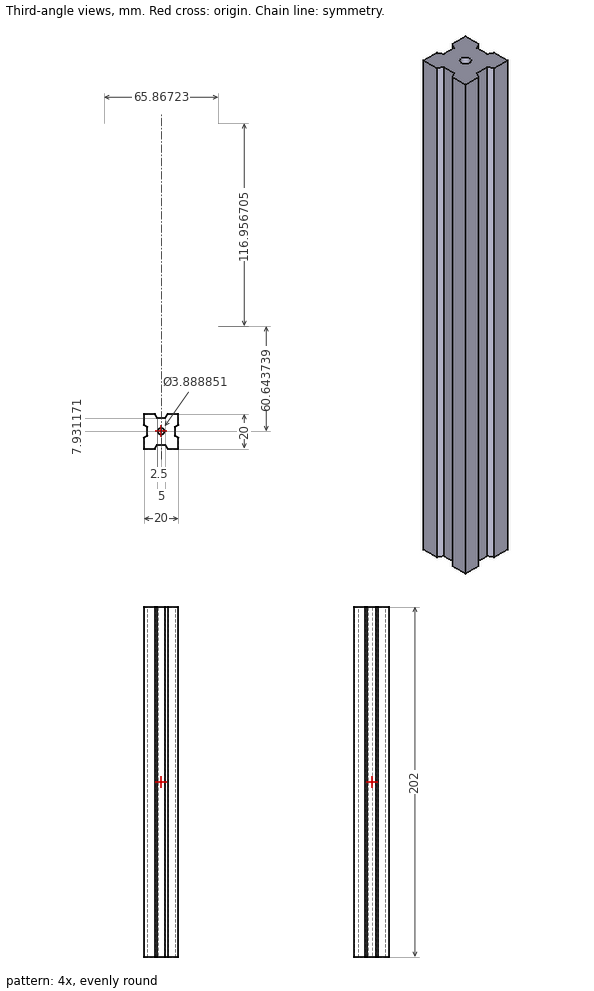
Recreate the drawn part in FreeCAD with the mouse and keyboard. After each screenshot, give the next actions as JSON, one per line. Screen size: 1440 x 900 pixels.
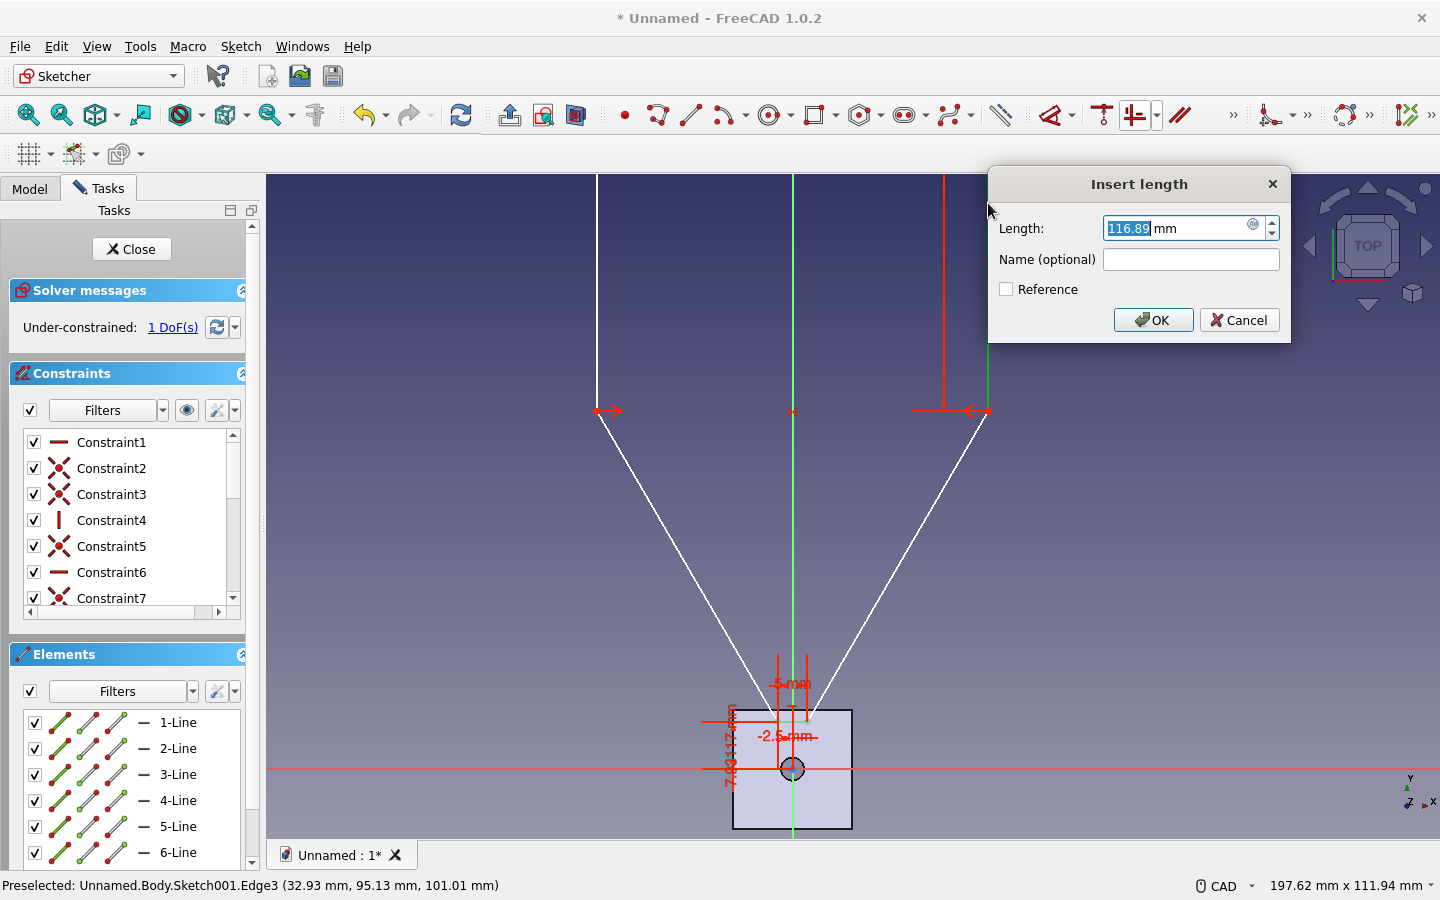
{"action": "type", "text": "116.956705"}
{"action": "key", "text": "Return"}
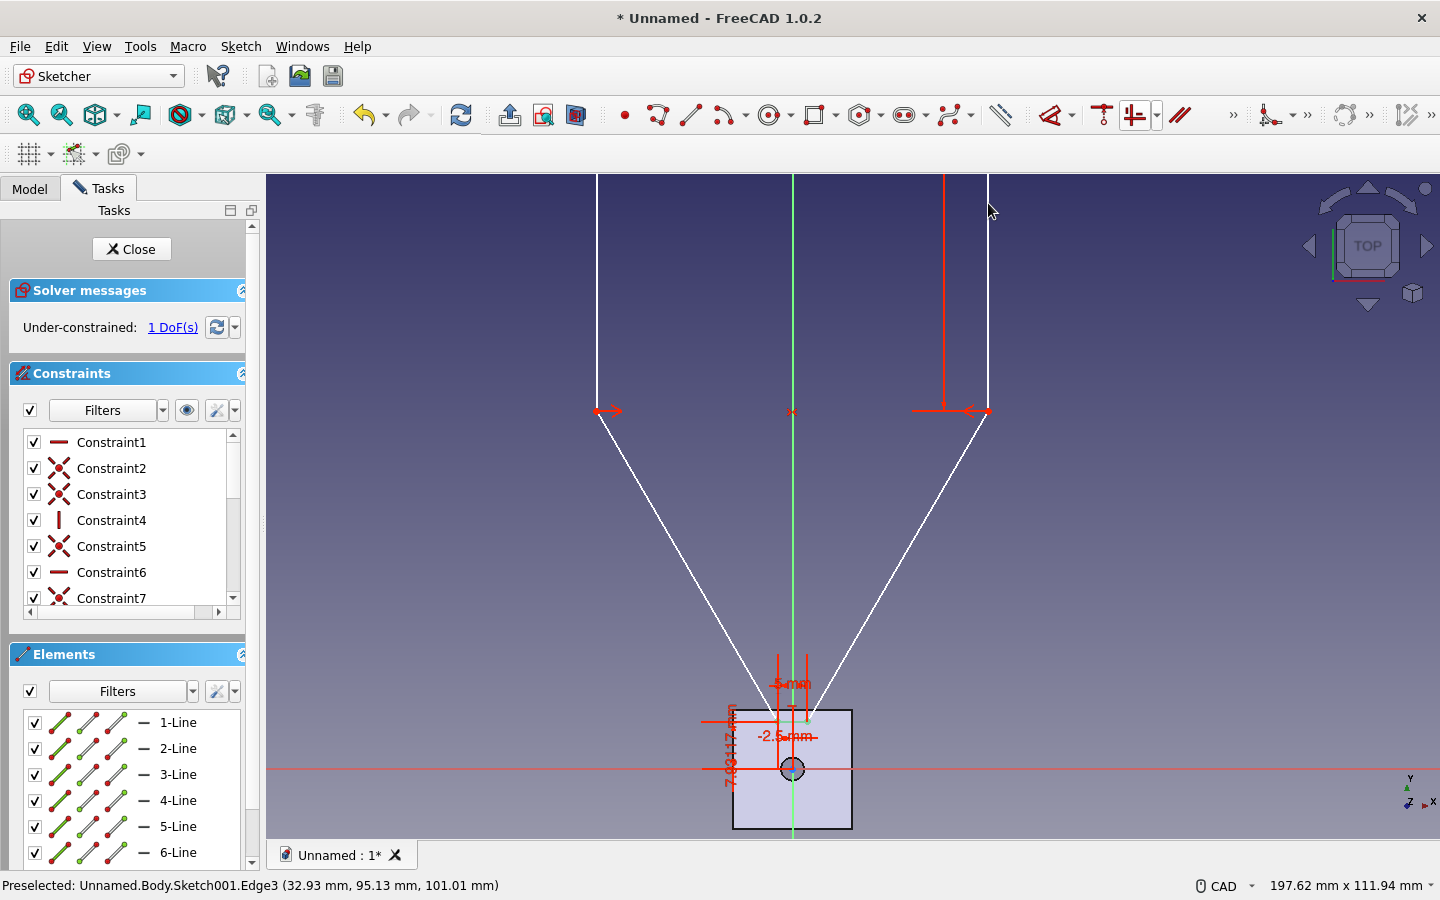
{"action": "left_click", "coordinate": [988, 411]}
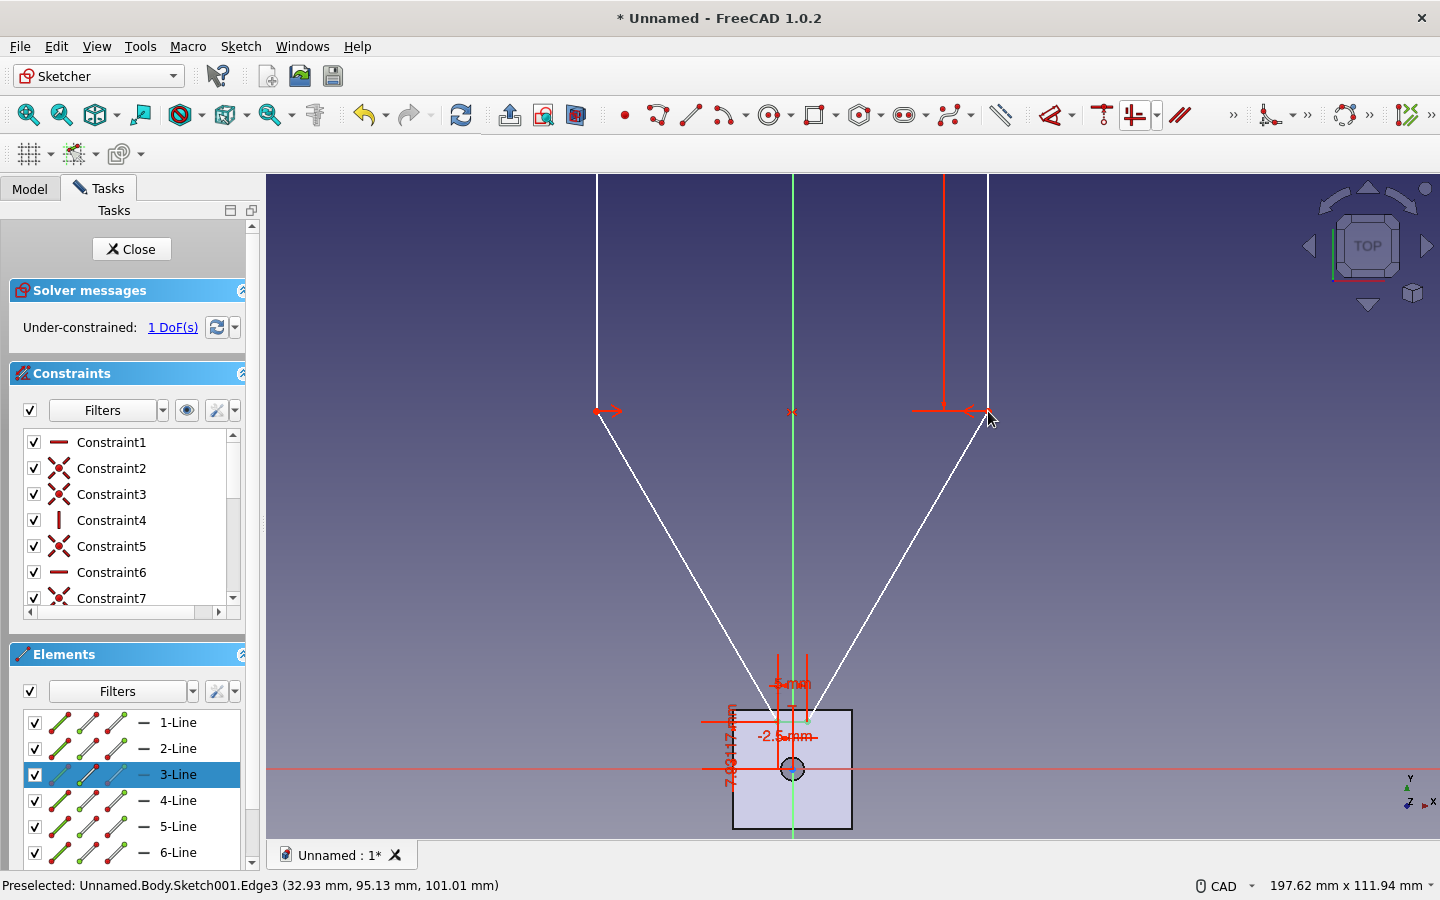
{"action": "key", "text": "i"}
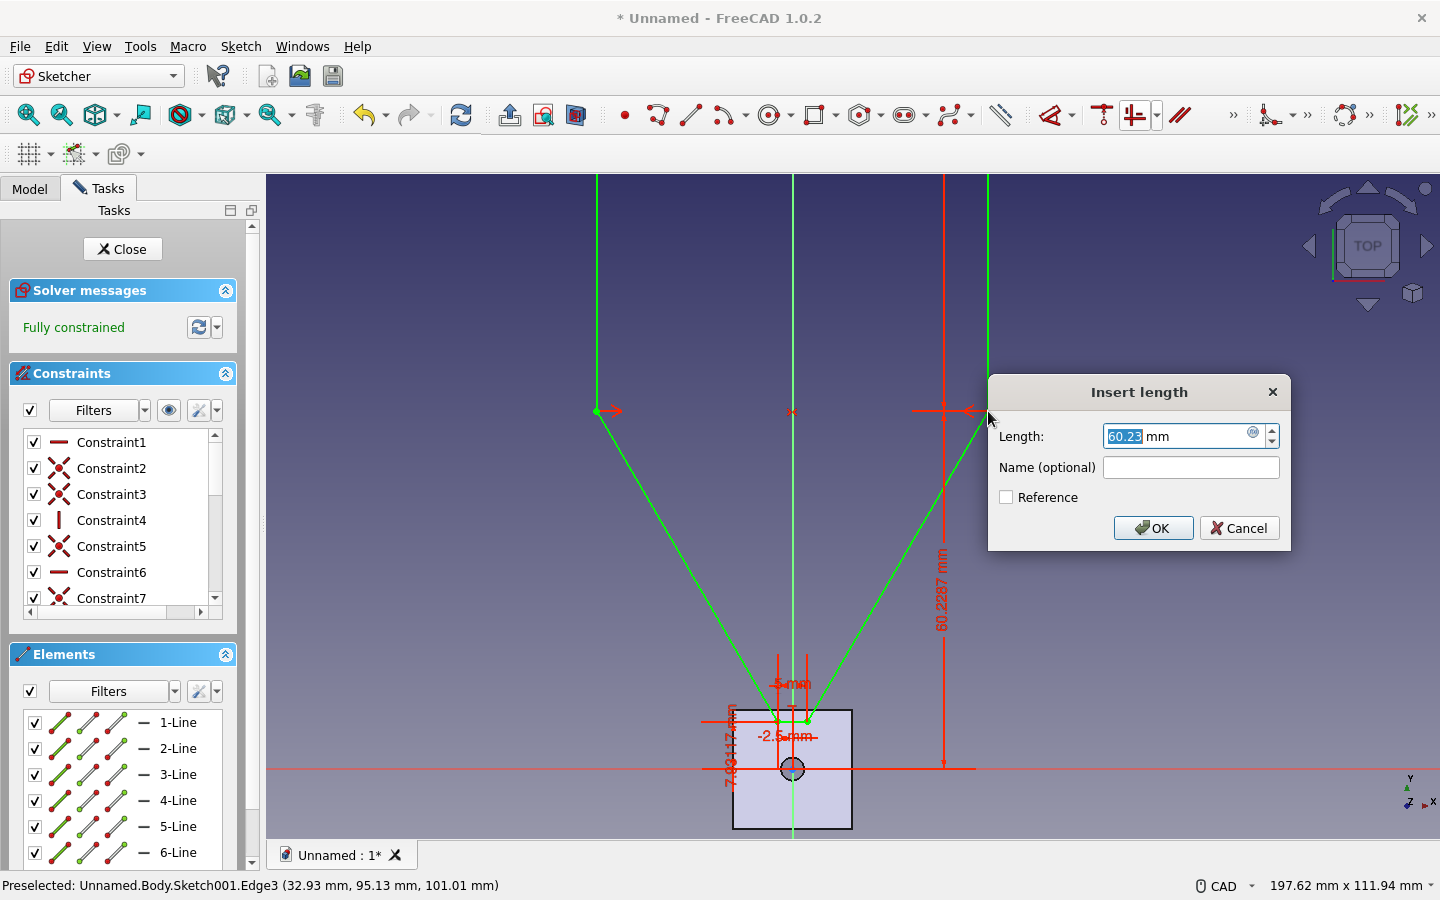
{"action": "type", "text": "60.643739"}
{"action": "key", "text": "Return"}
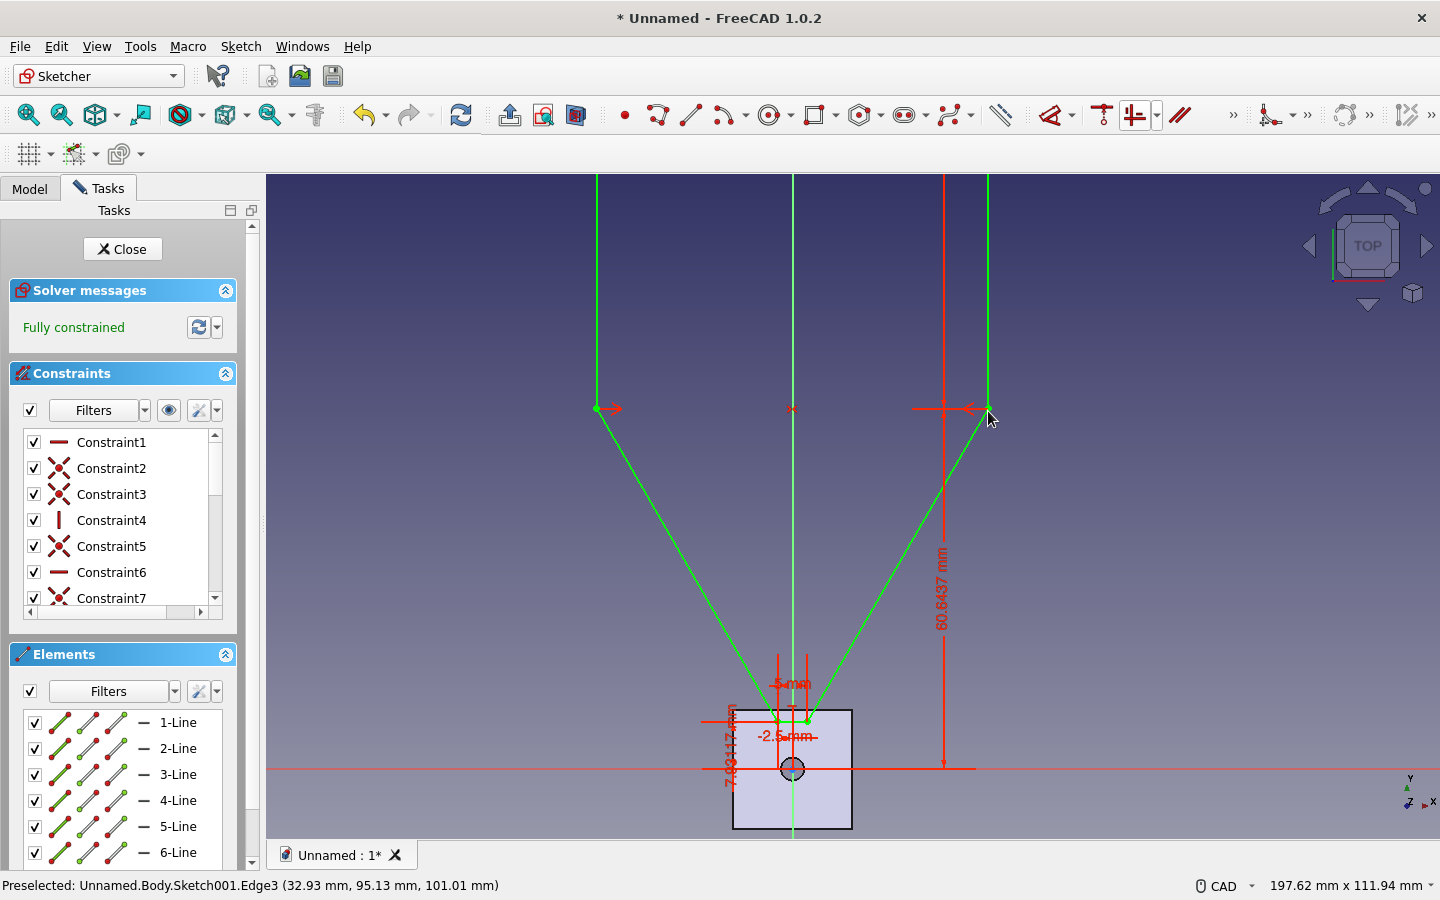
{"action": "left_click", "coordinate": [123, 249]}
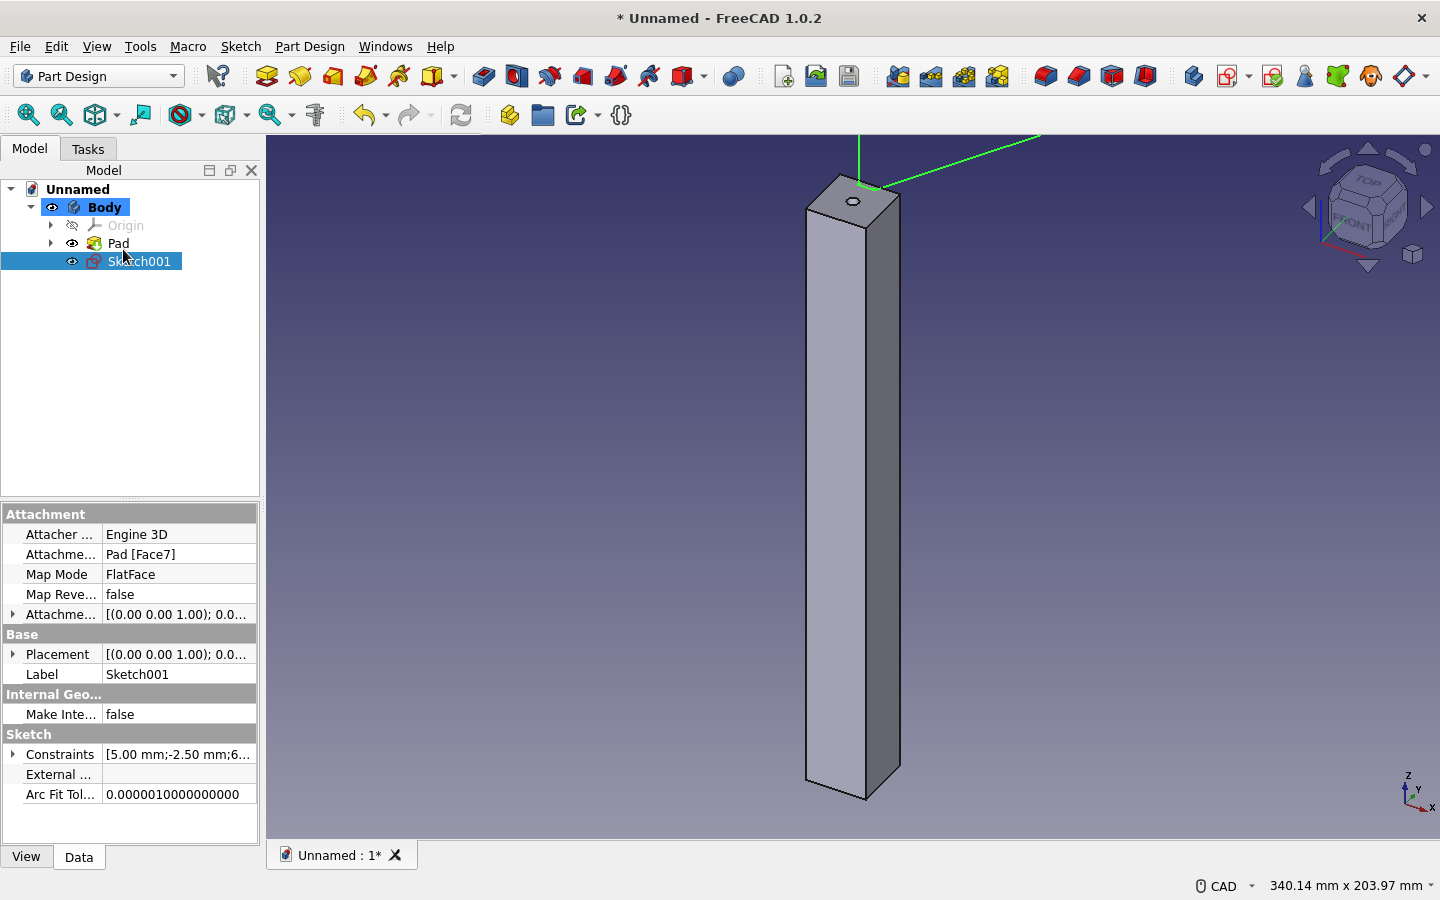
{"action": "left_click", "coordinate": [484, 76]}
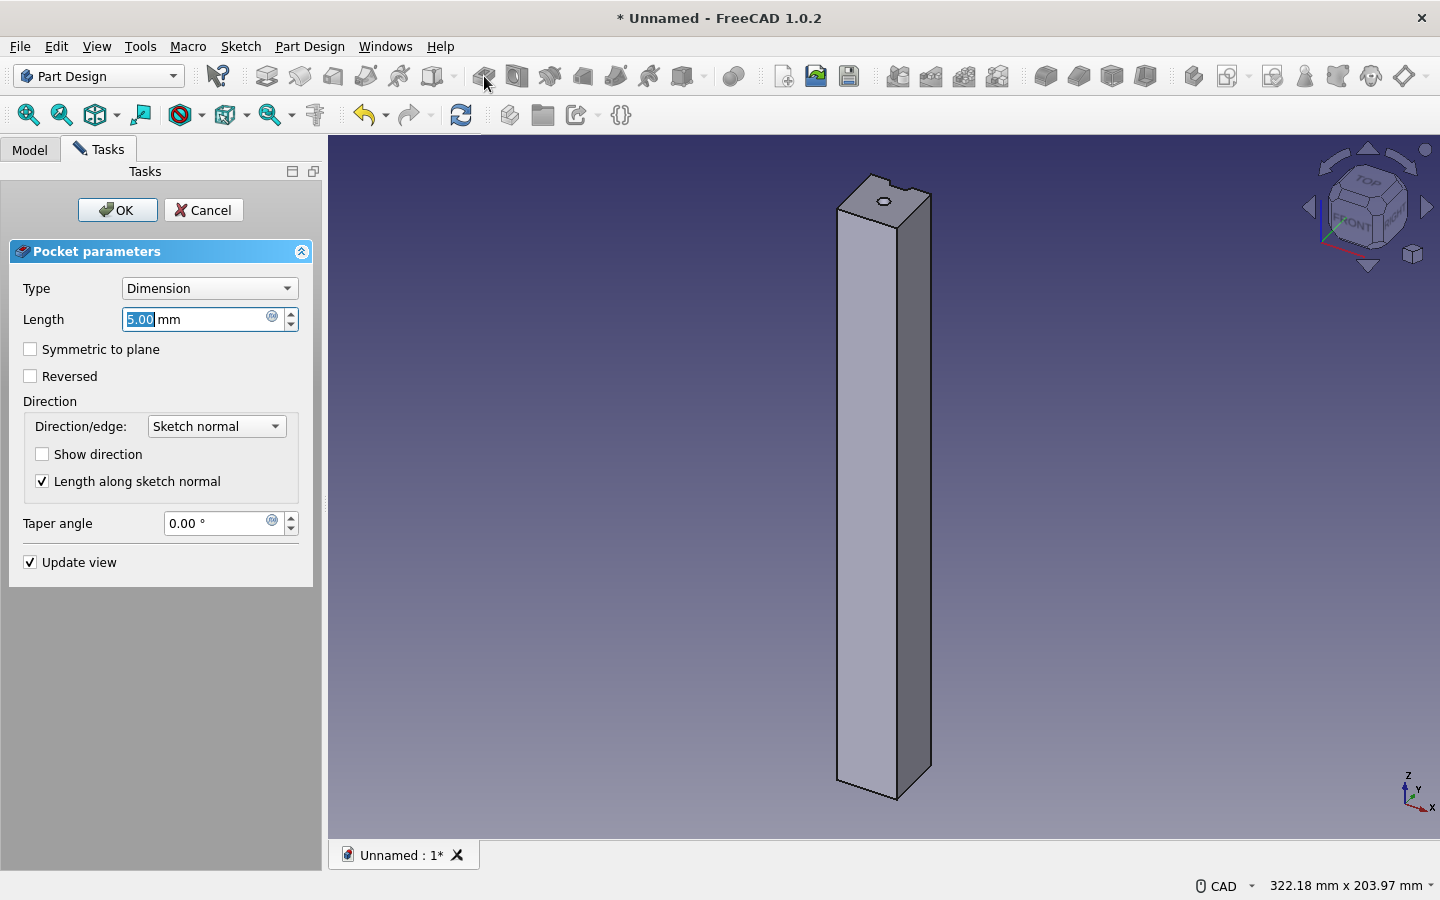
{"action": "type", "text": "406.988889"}
{"action": "key", "text": "Tab"}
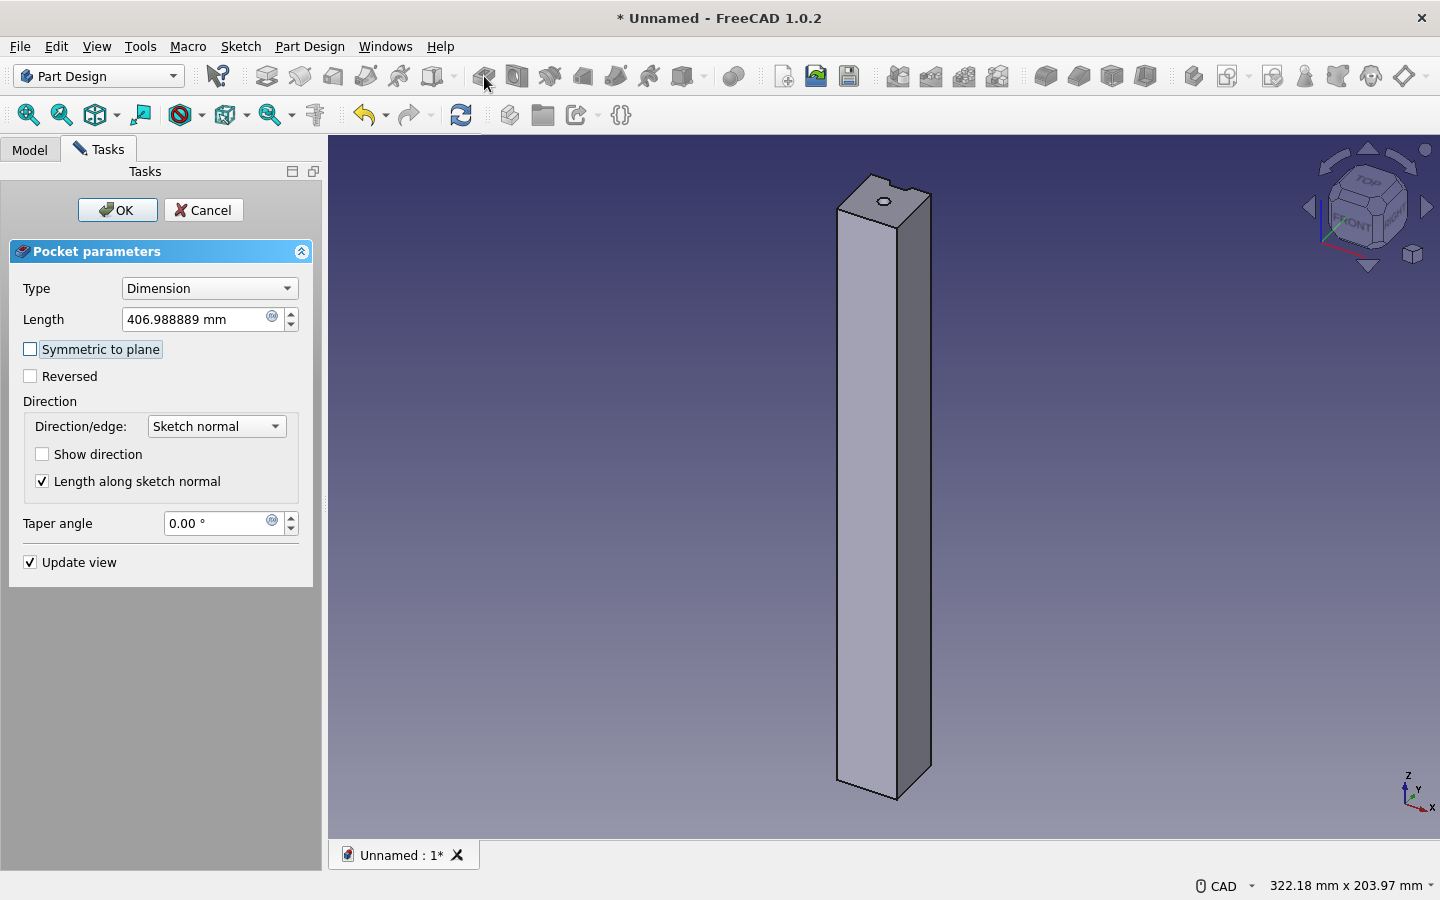
{"action": "left_click", "coordinate": [31, 349]}